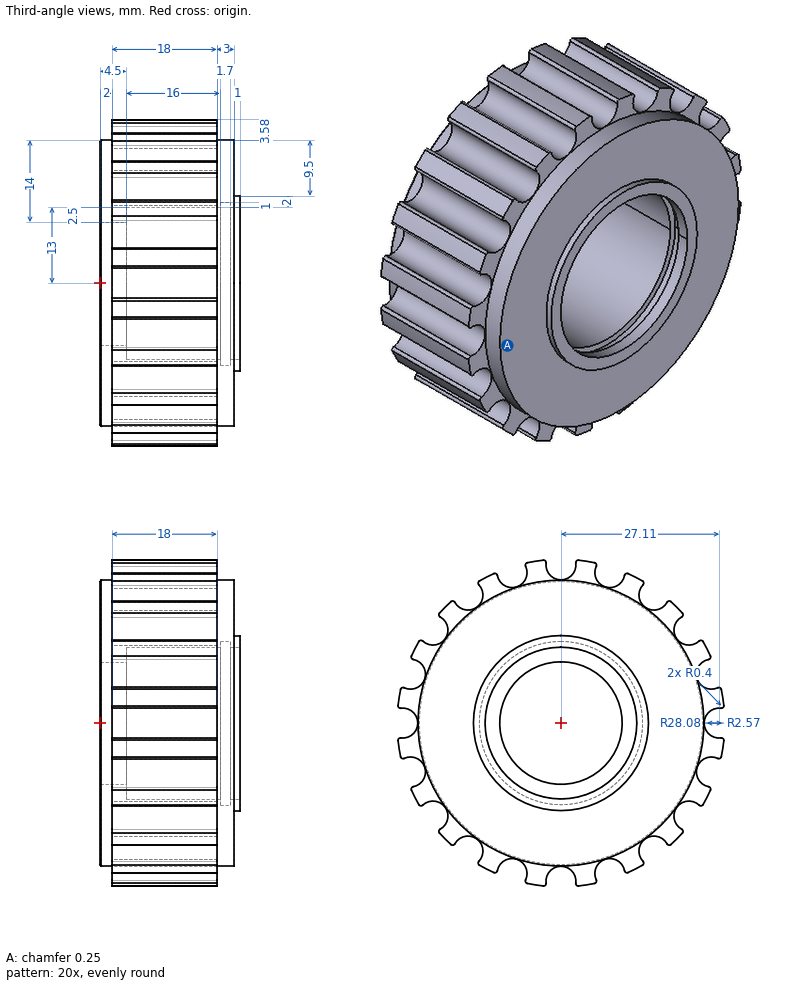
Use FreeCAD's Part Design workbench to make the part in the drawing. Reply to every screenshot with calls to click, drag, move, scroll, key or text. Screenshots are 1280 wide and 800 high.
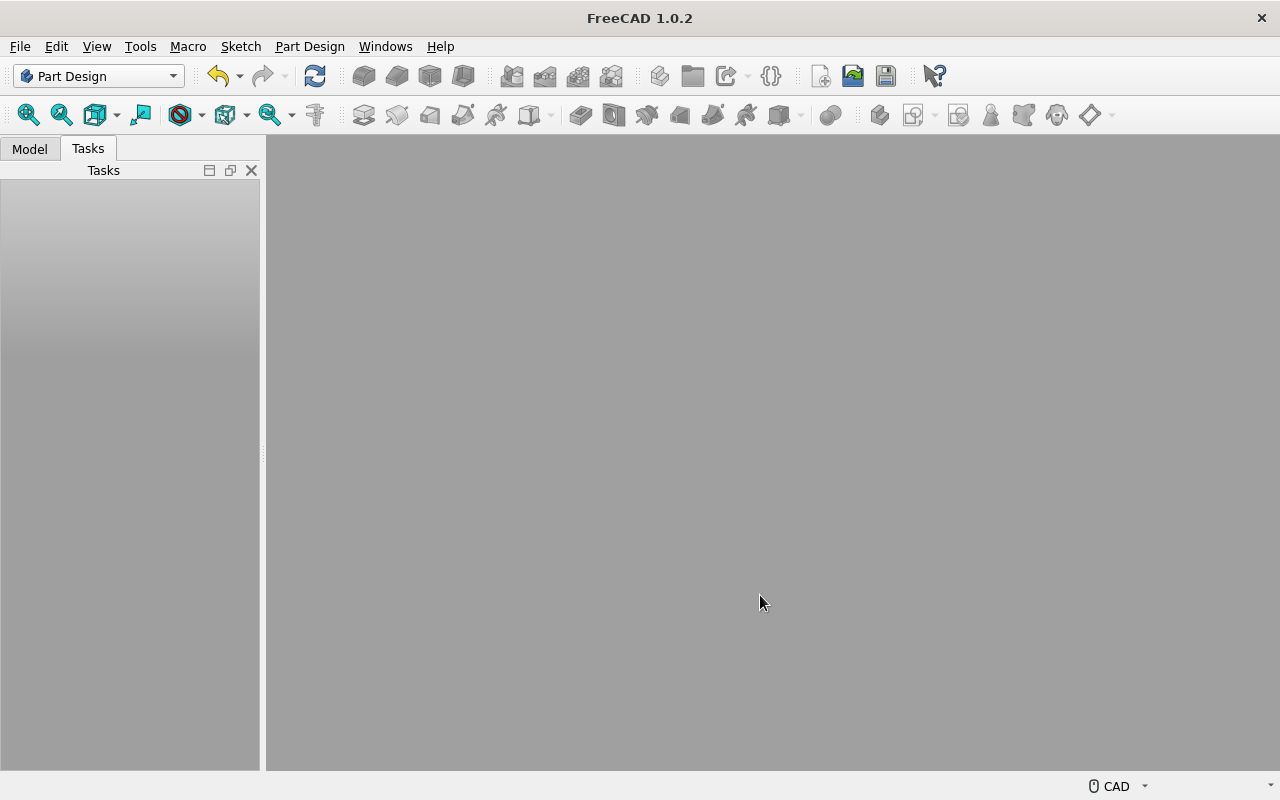
click(820, 76)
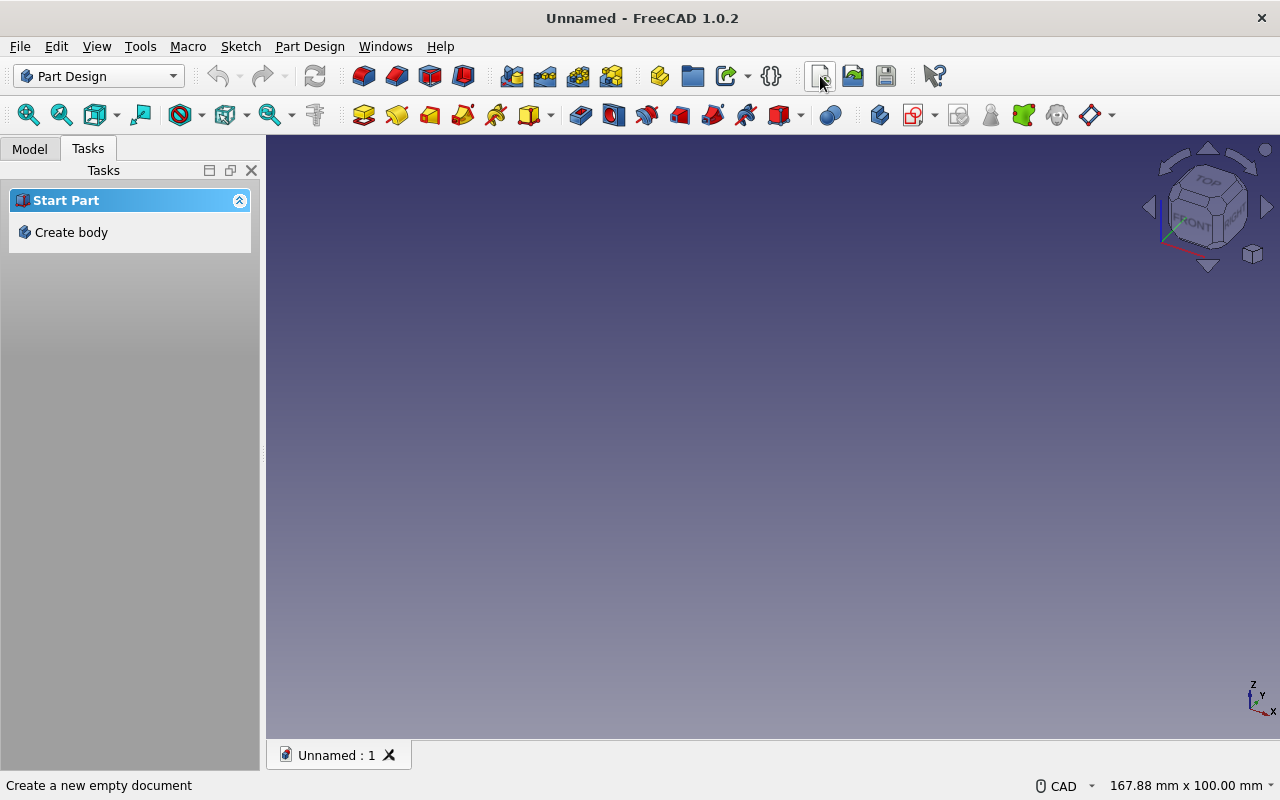
click(912, 116)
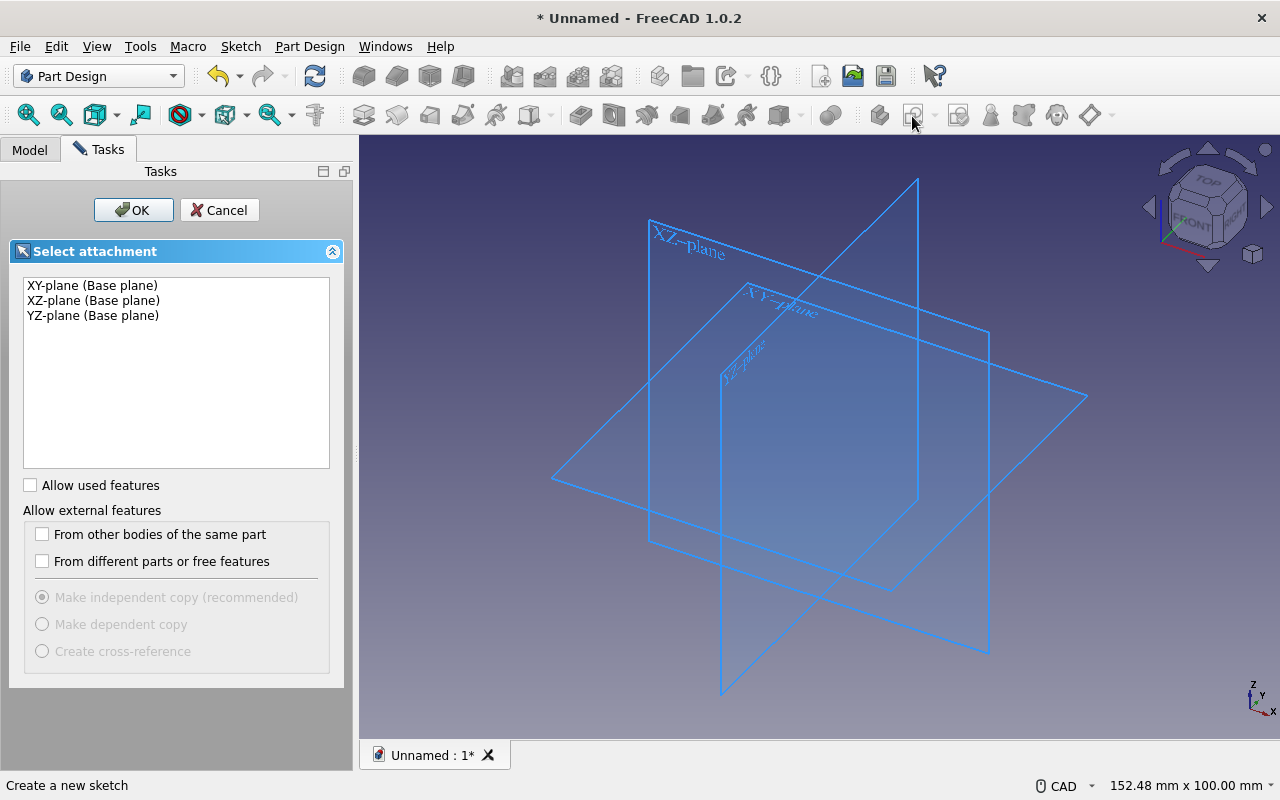
click(84, 286)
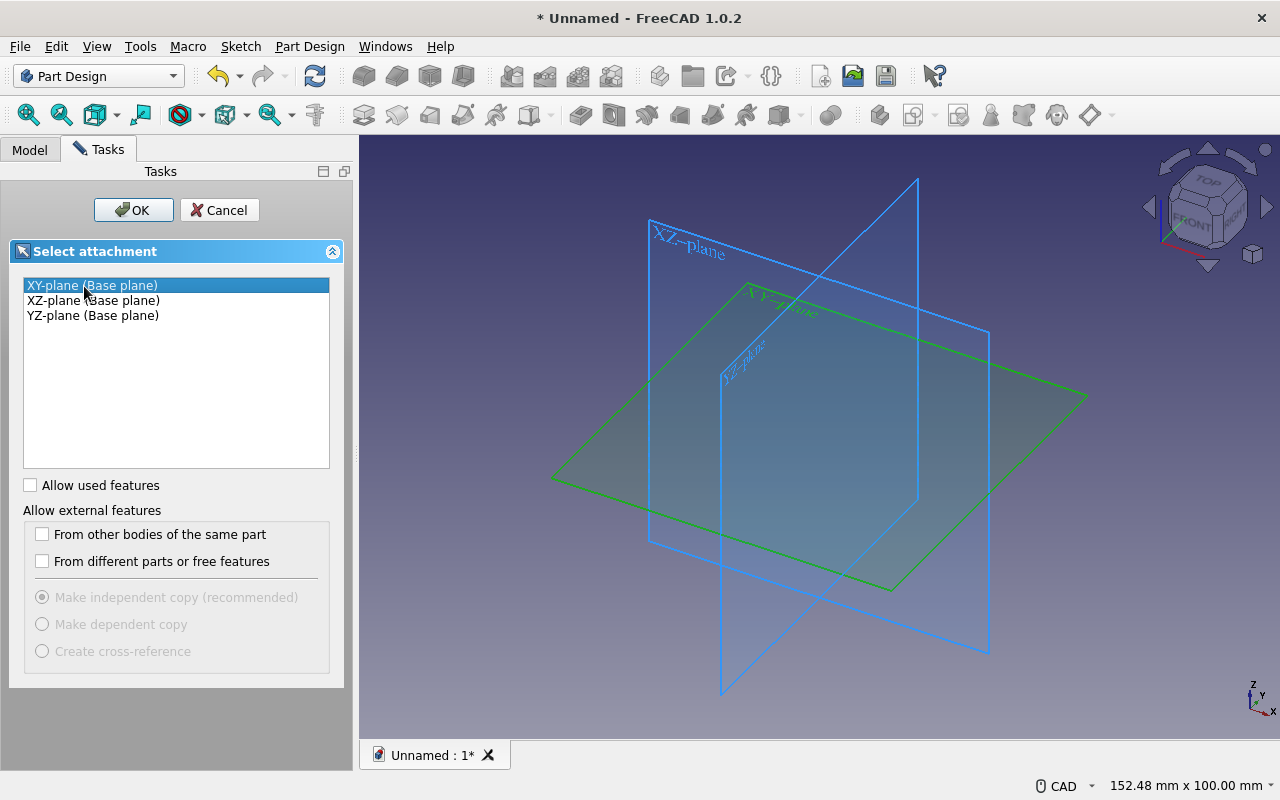
click(134, 210)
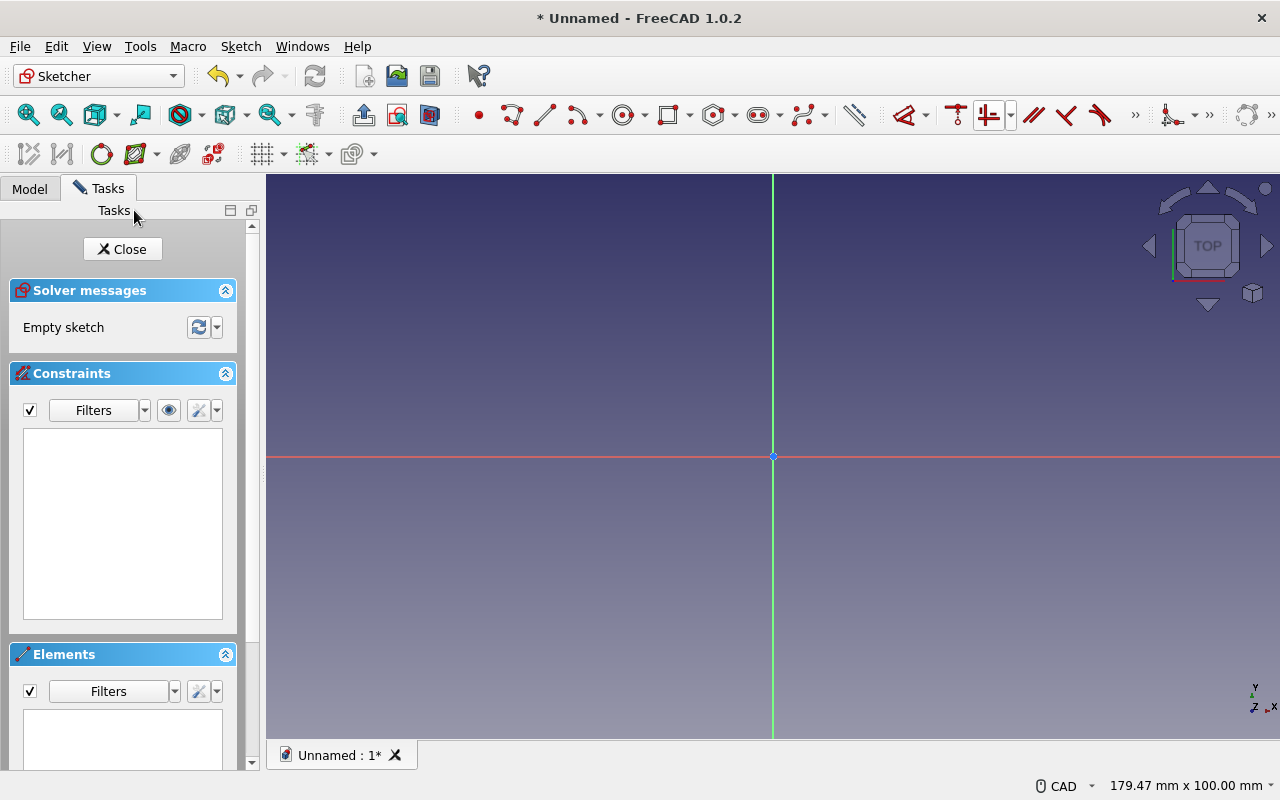
scroll(952, 312, up, 4)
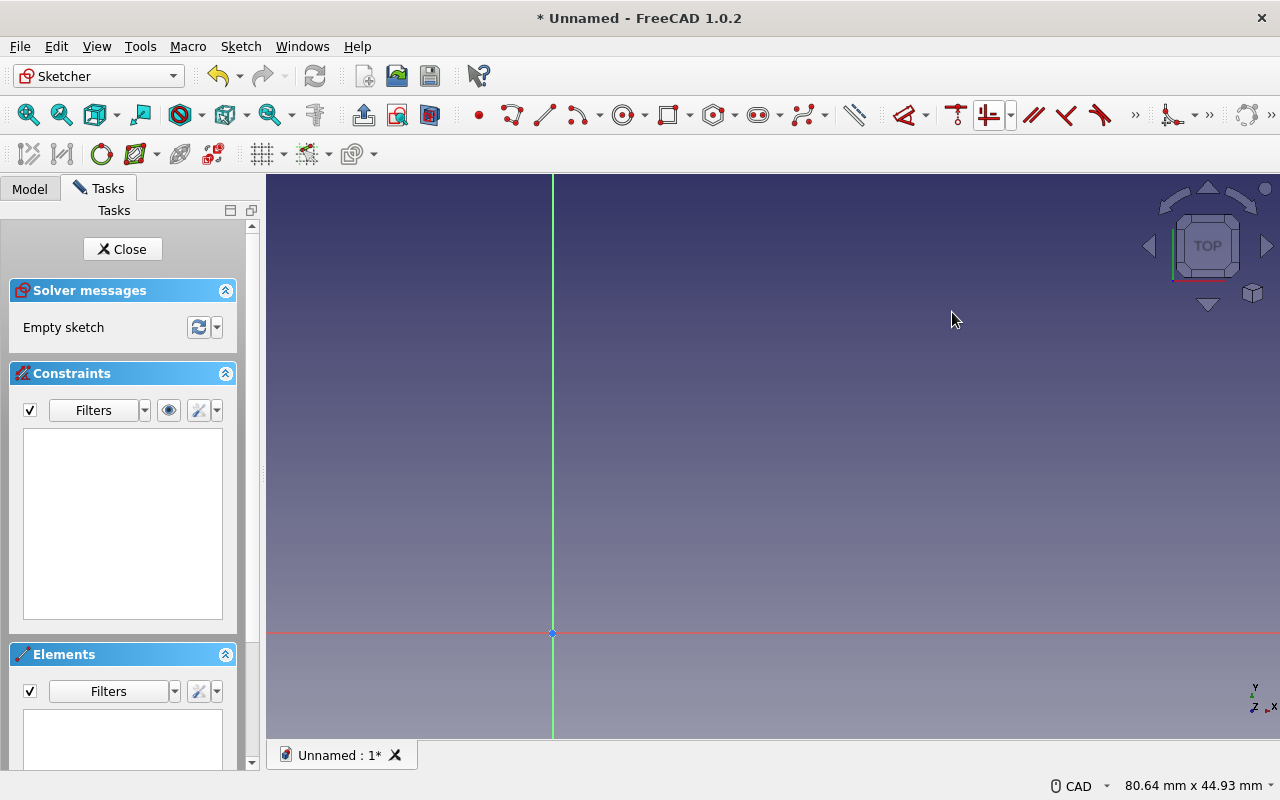
click(512, 116)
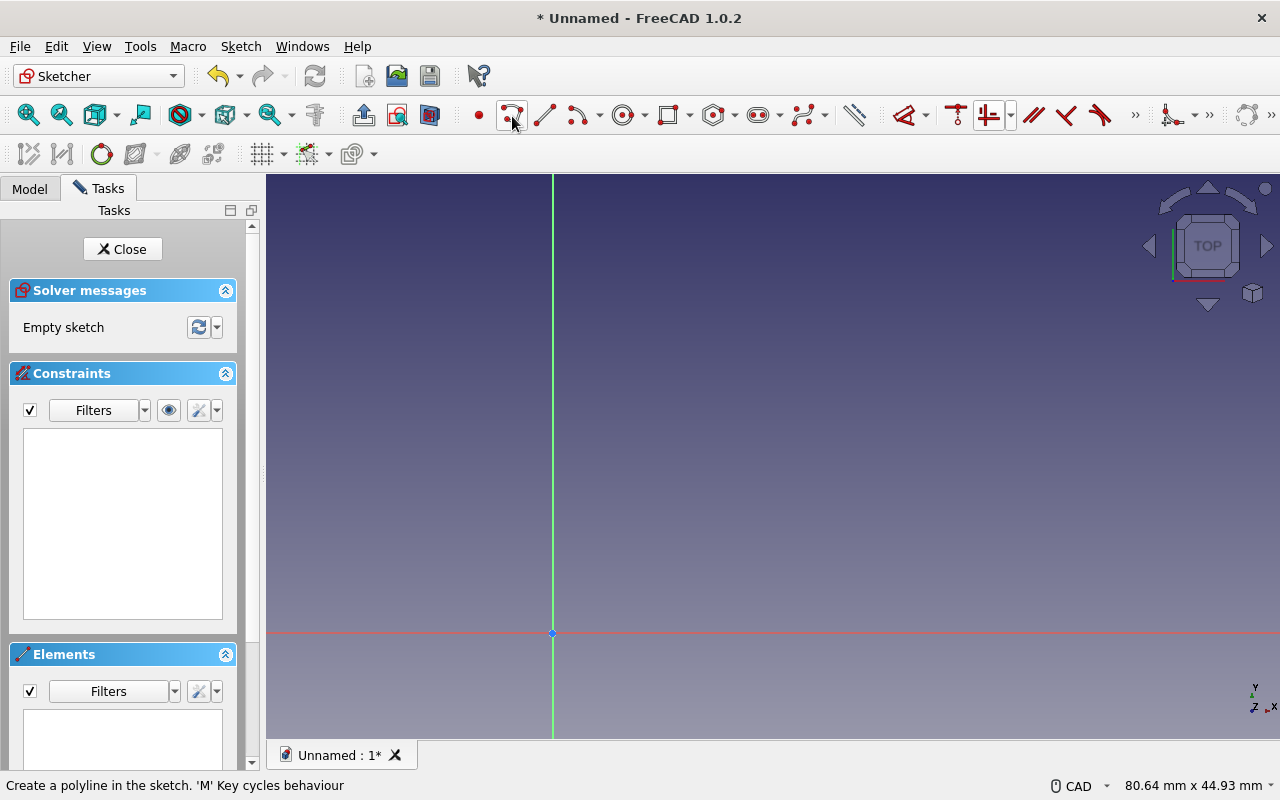
click(553, 501)
click(609, 501)
click(609, 470)
click(811, 470)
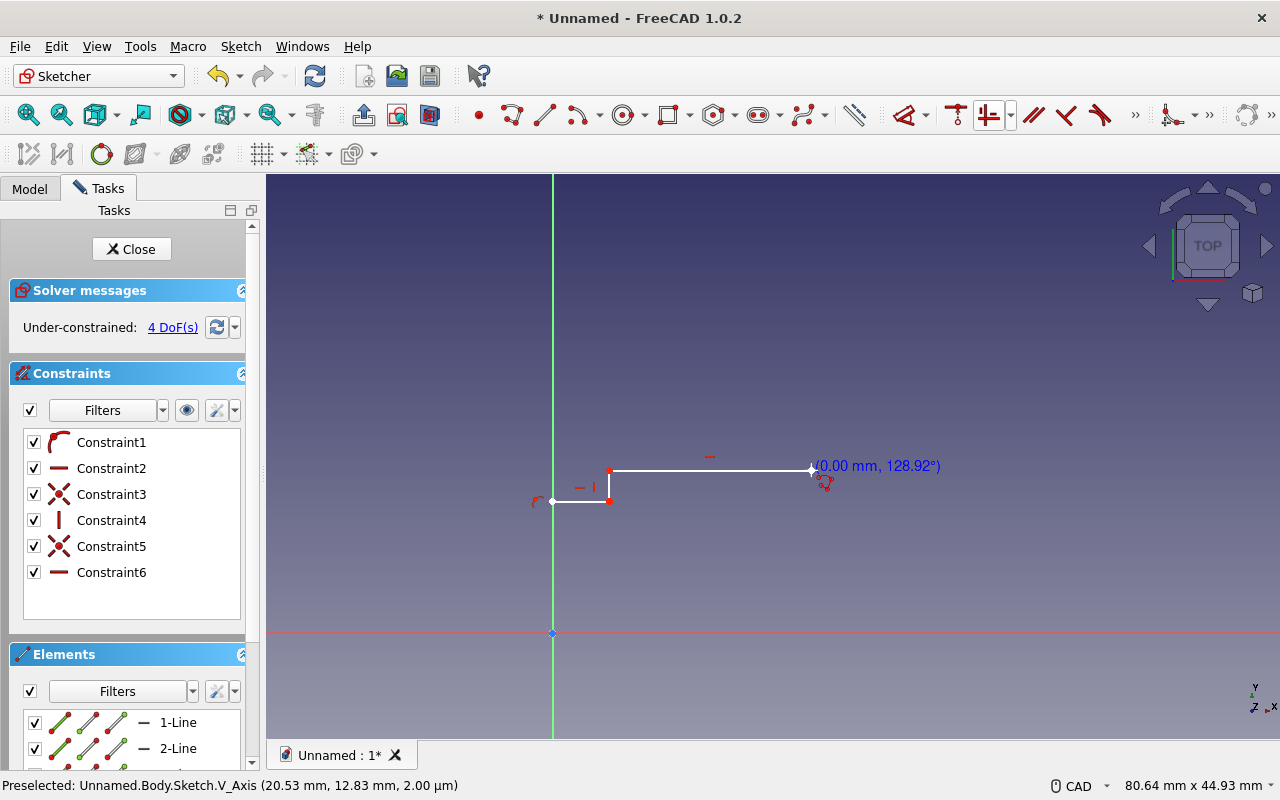
scroll(811, 457, up, 2)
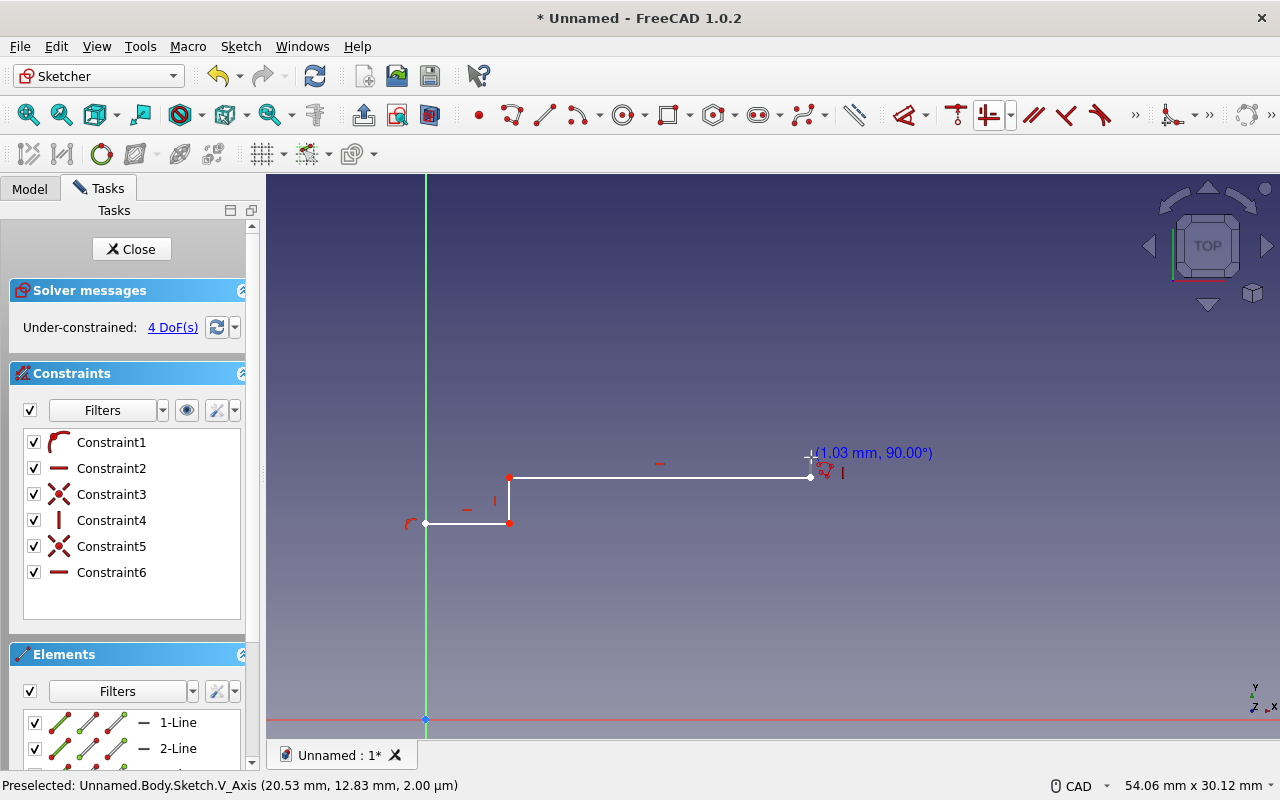
click(811, 457)
click(842, 457)
click(842, 476)
click(876, 476)
click(876, 438)
click(857, 438)
click(857, 260)
click(801, 260)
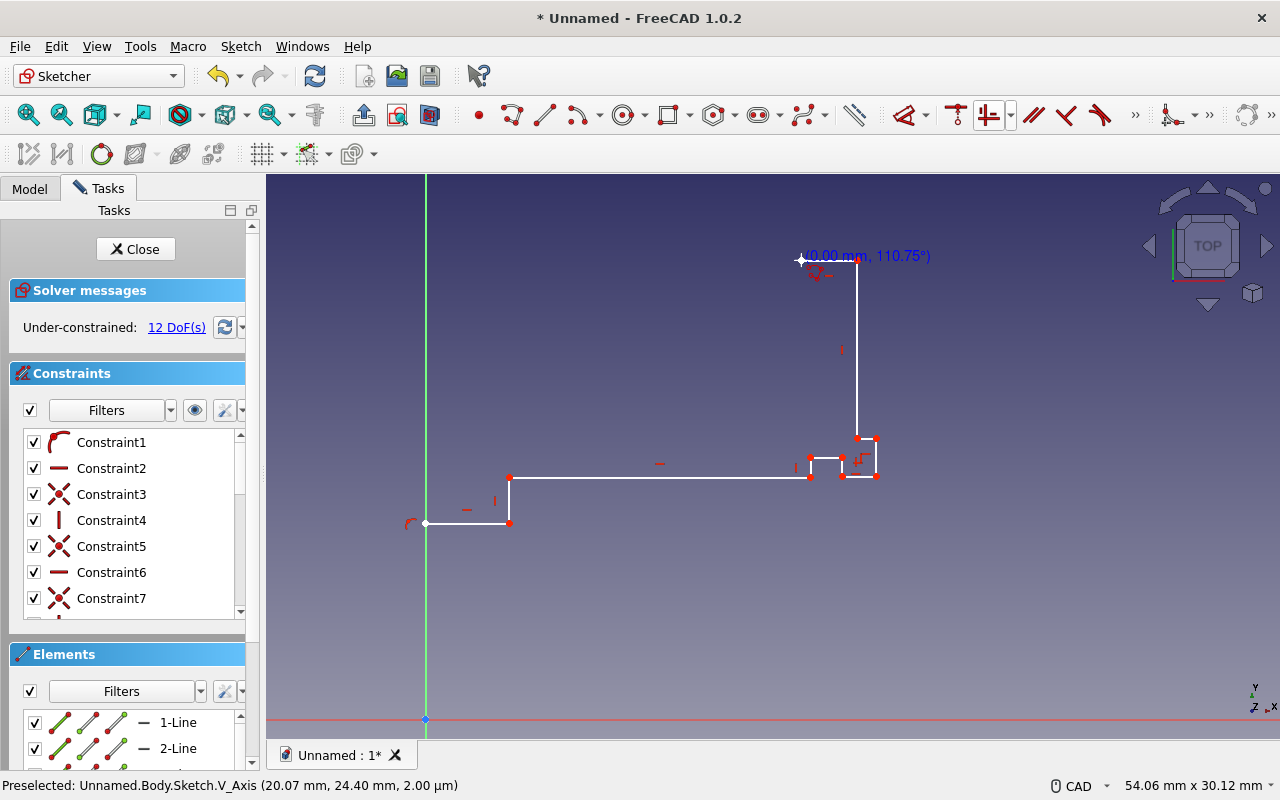
scroll(814, 457, down, 2)